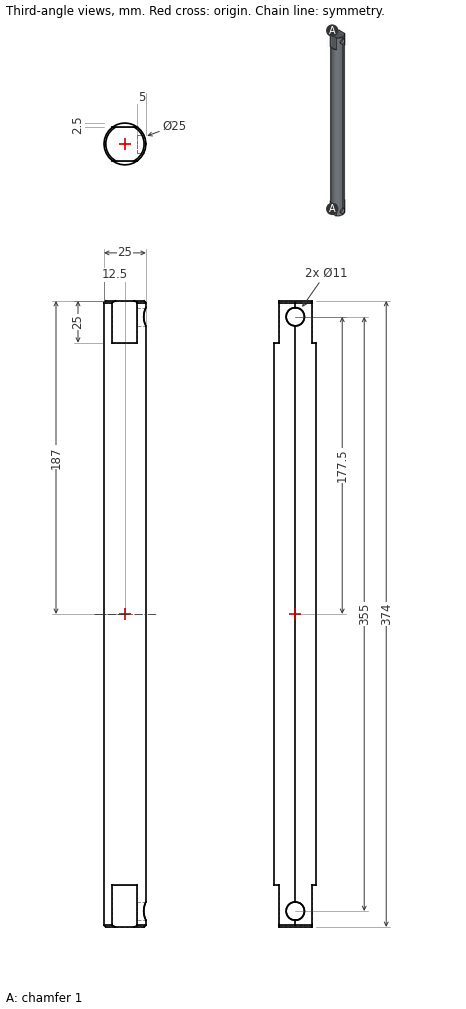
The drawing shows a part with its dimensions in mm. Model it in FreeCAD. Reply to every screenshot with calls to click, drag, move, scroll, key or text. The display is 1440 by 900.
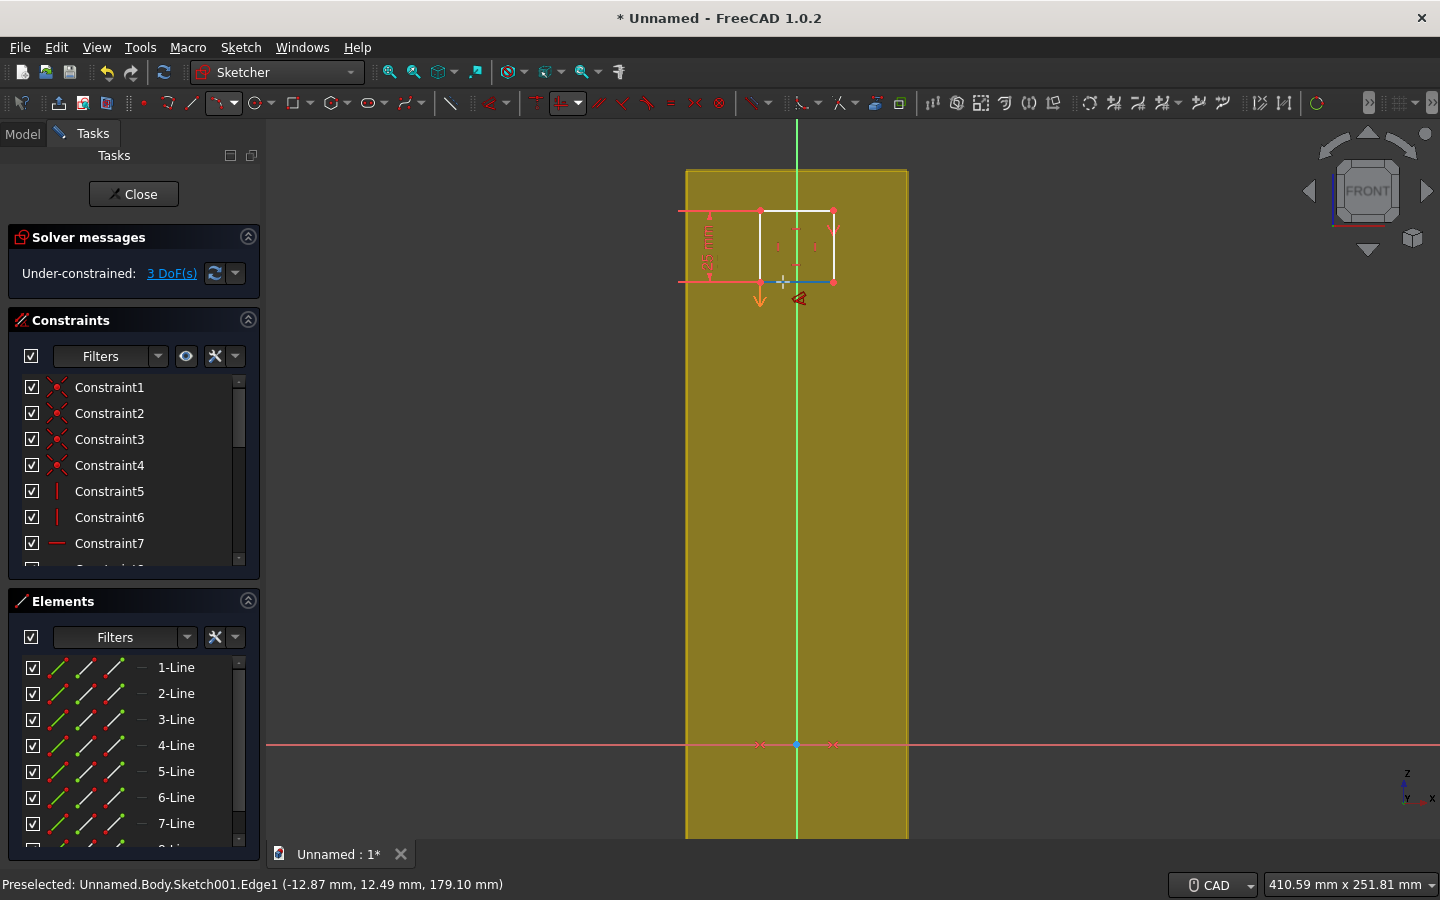
click(782, 282)
click(780, 248)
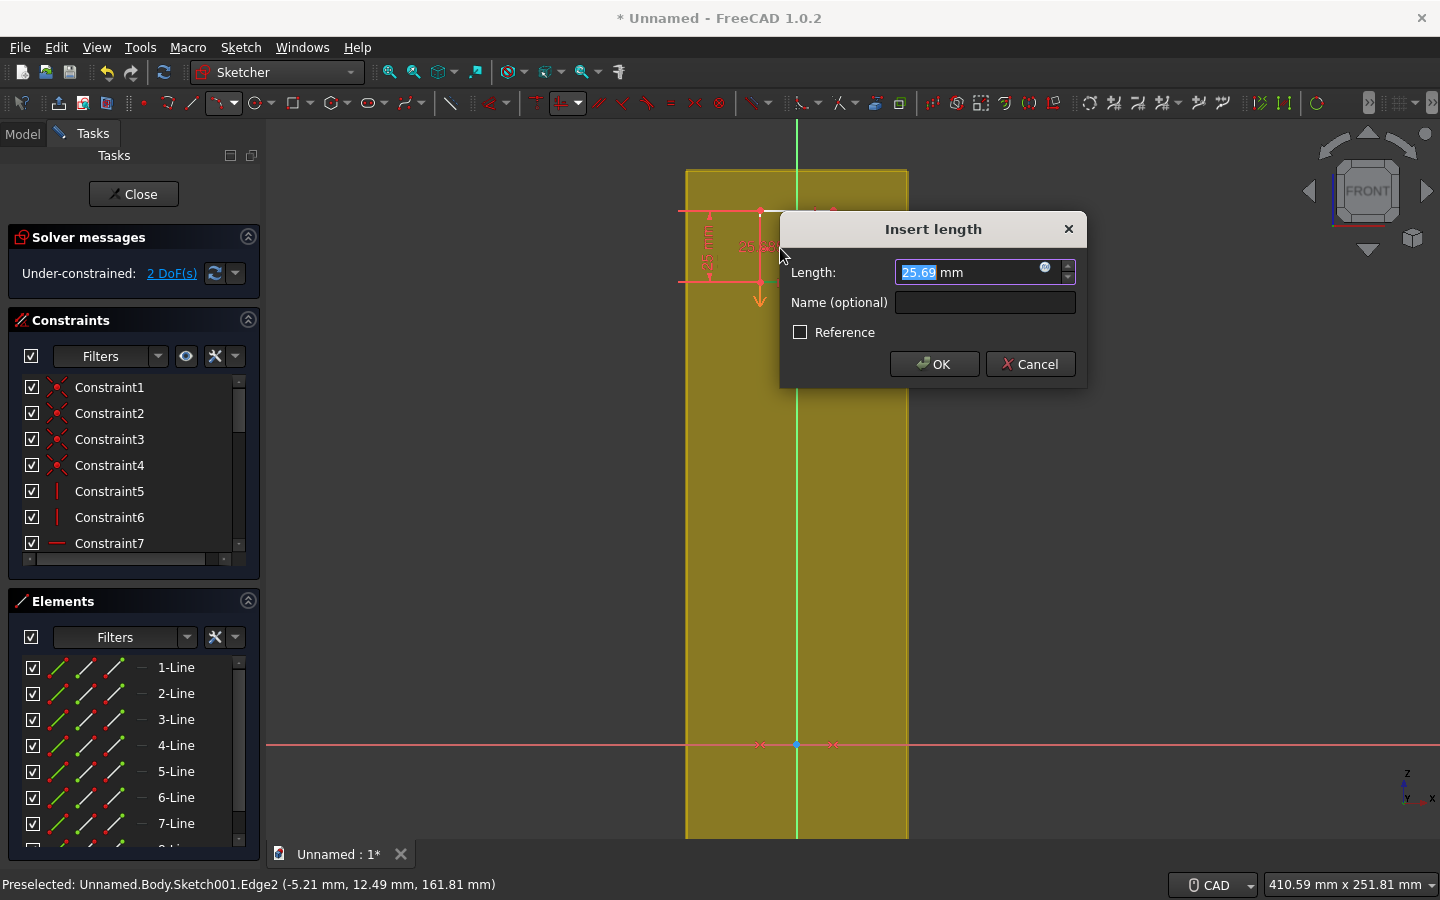
text(25)
key(Return)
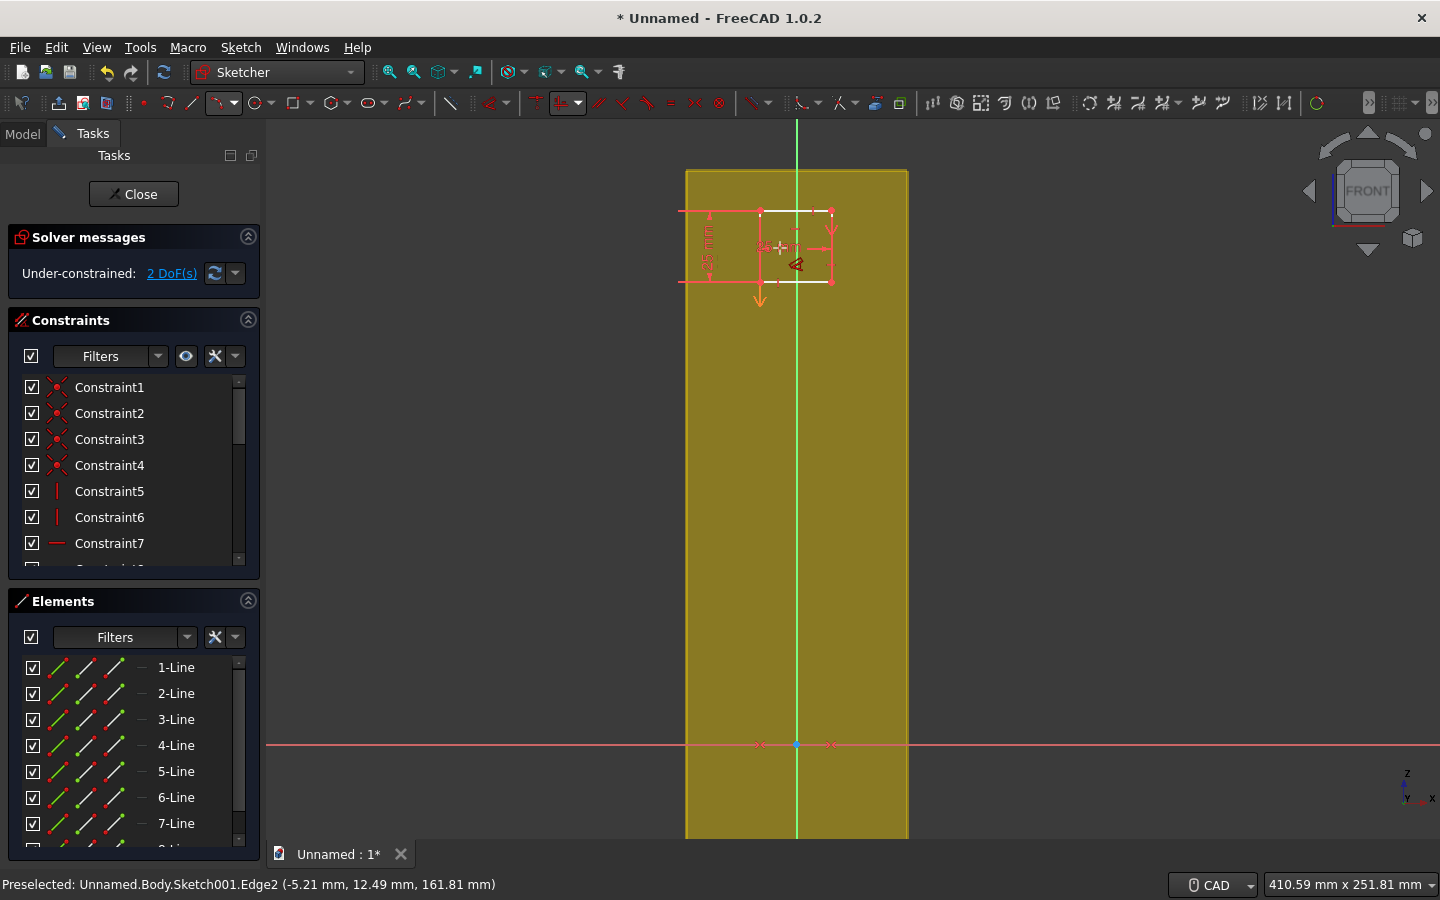
click(760, 211)
click(726, 478)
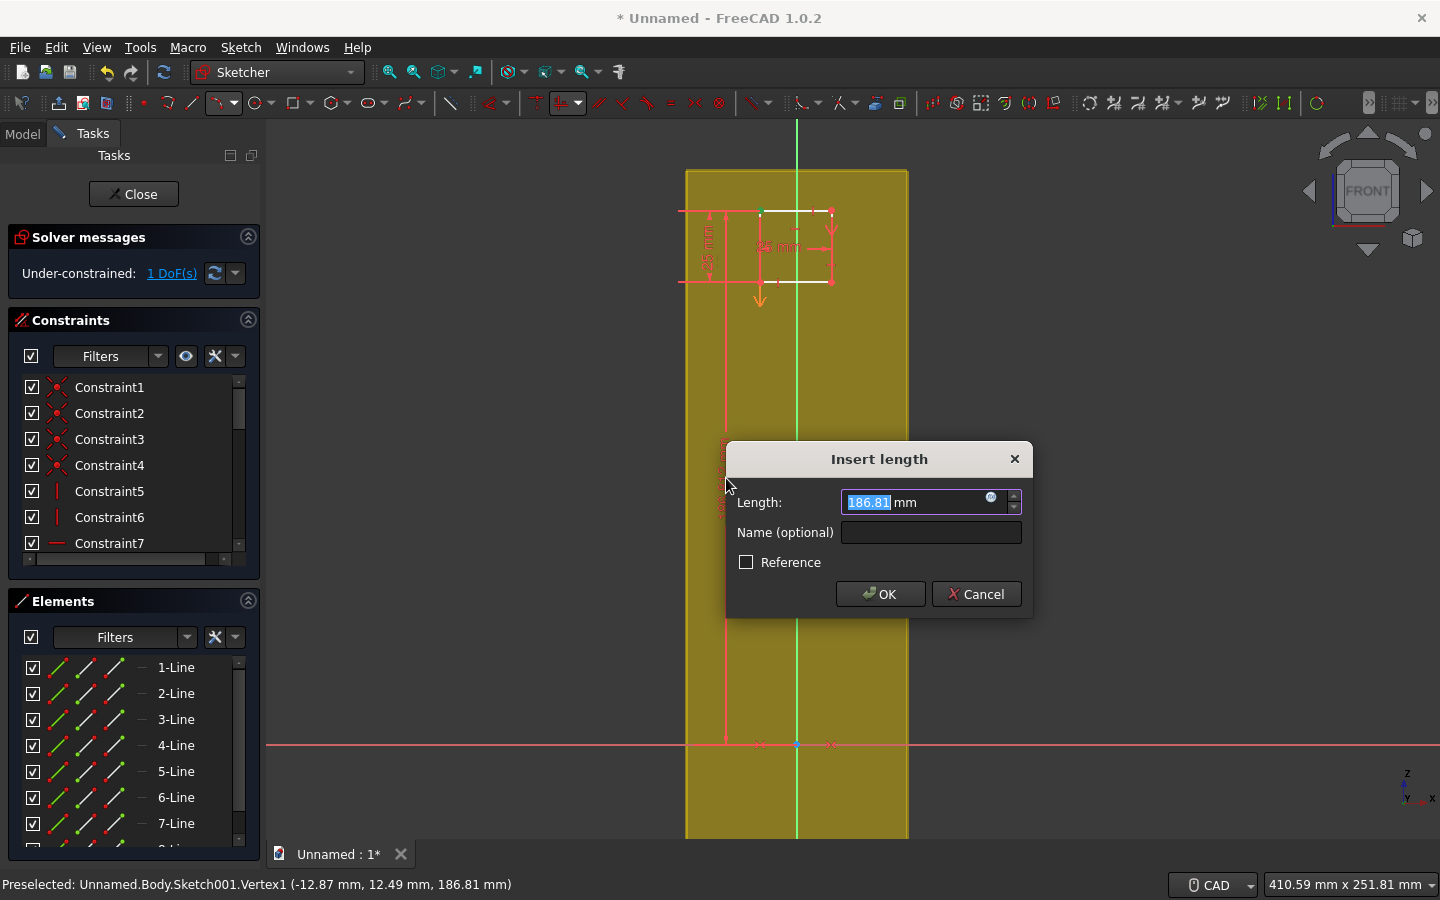
text(187)
key(Return)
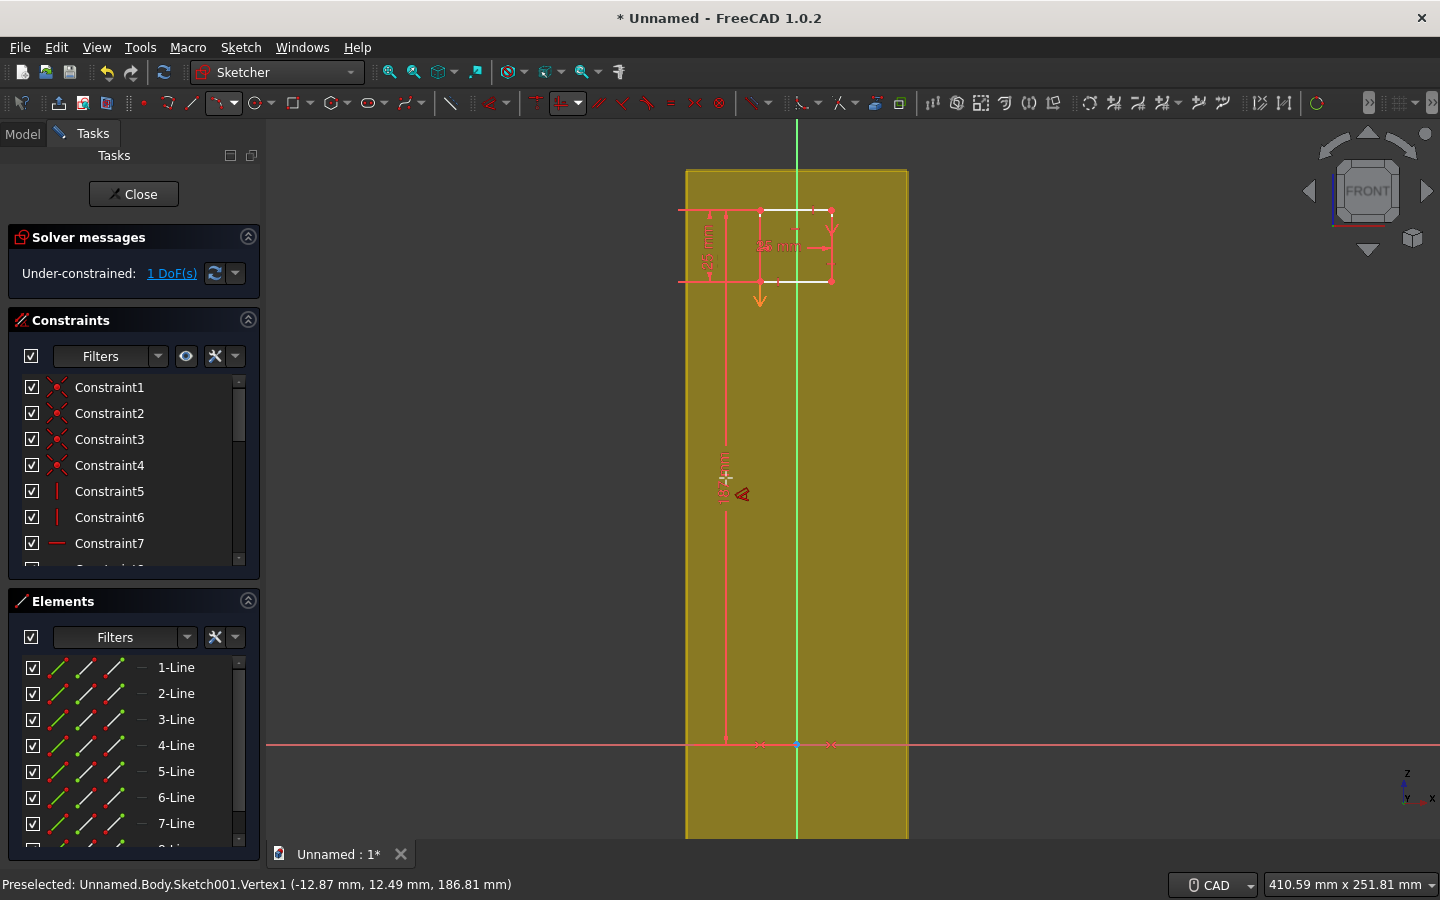
click(760, 210)
click(778, 176)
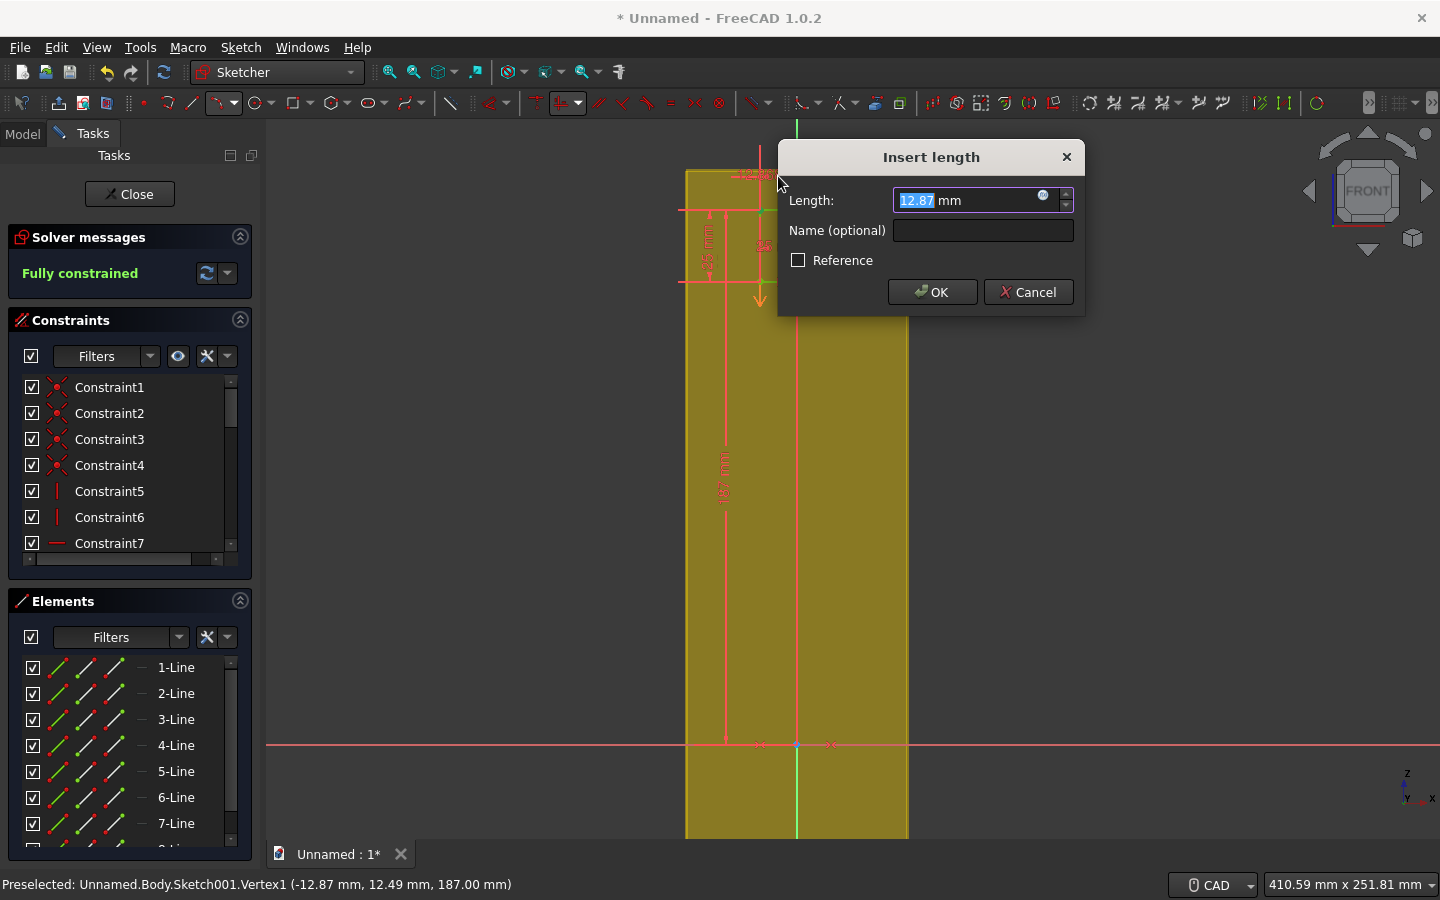
text(12.5)
key(Return)
key(Escape)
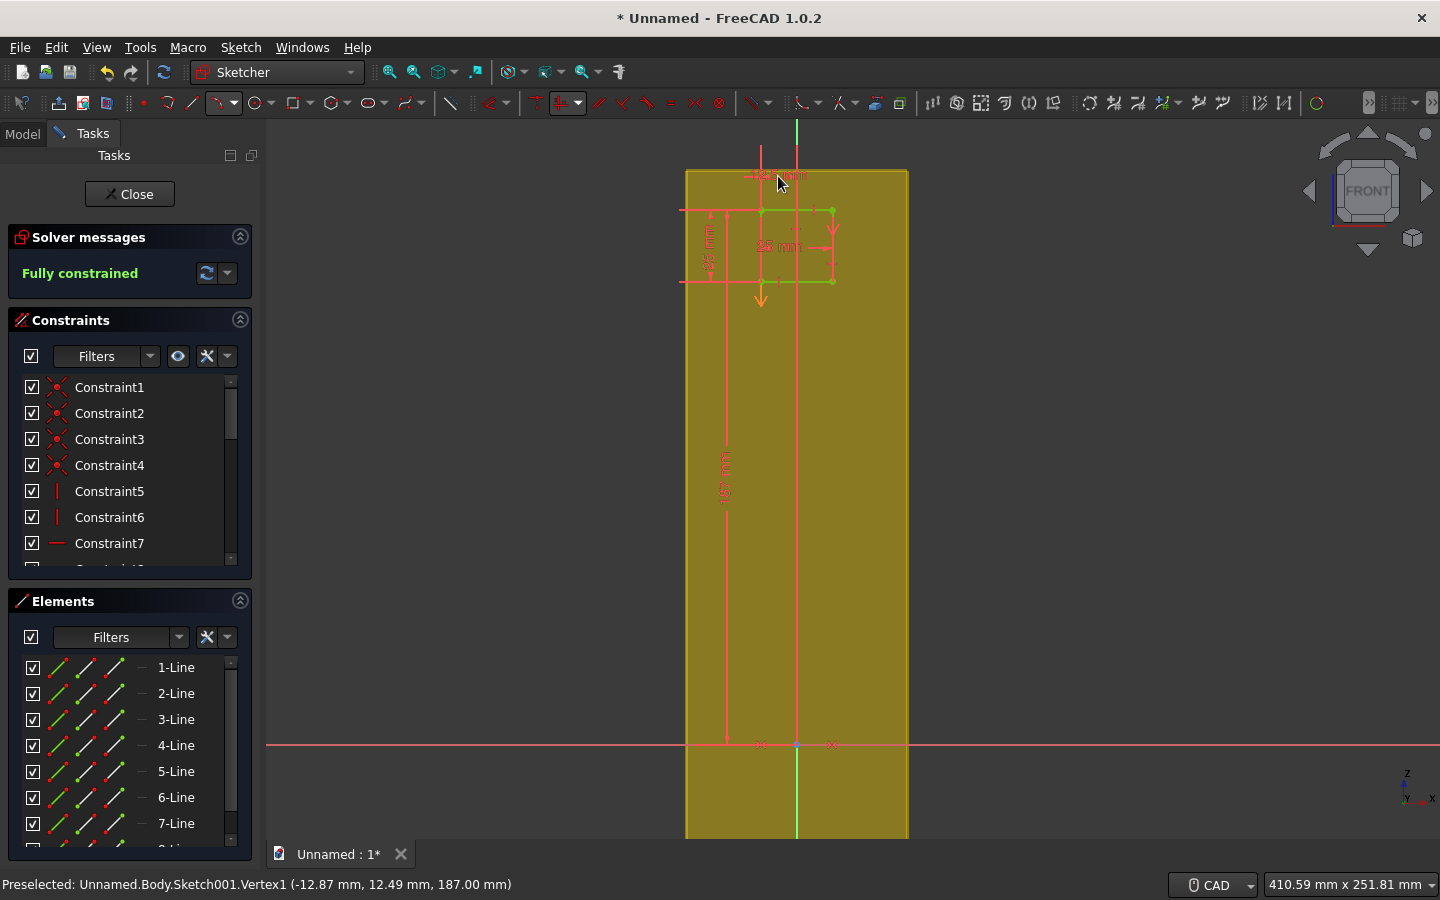
click(130, 194)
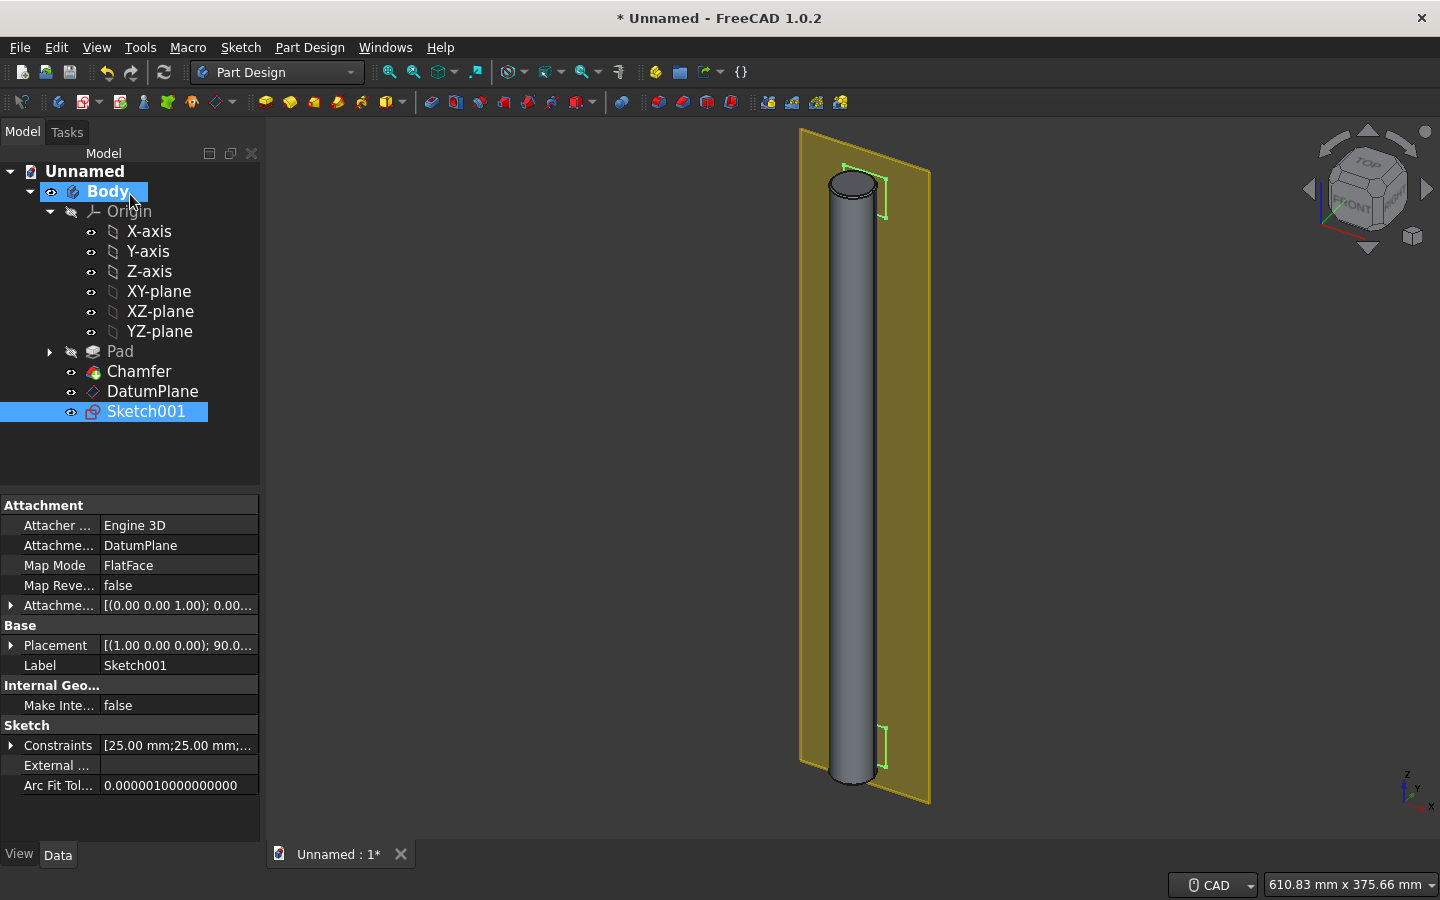
click(432, 102)